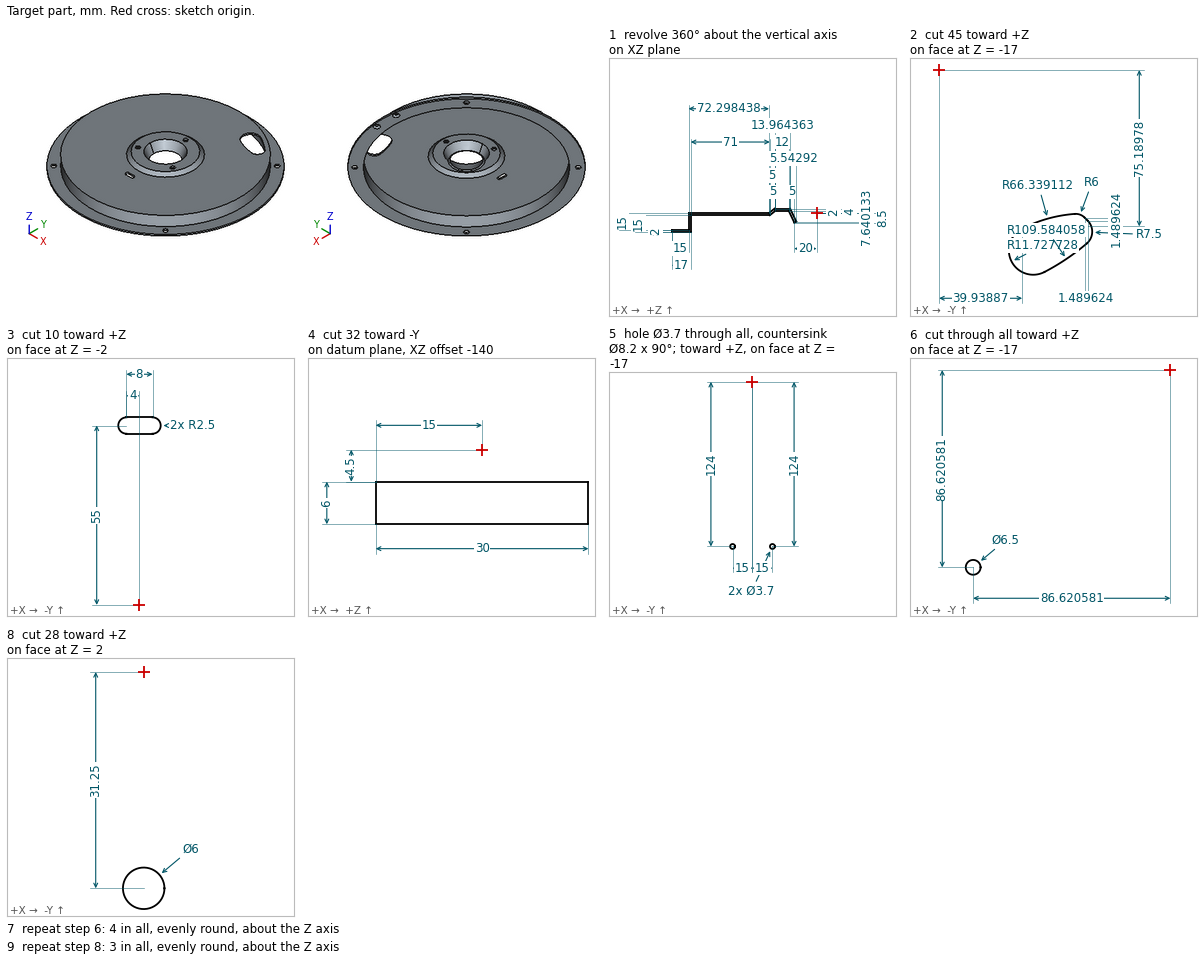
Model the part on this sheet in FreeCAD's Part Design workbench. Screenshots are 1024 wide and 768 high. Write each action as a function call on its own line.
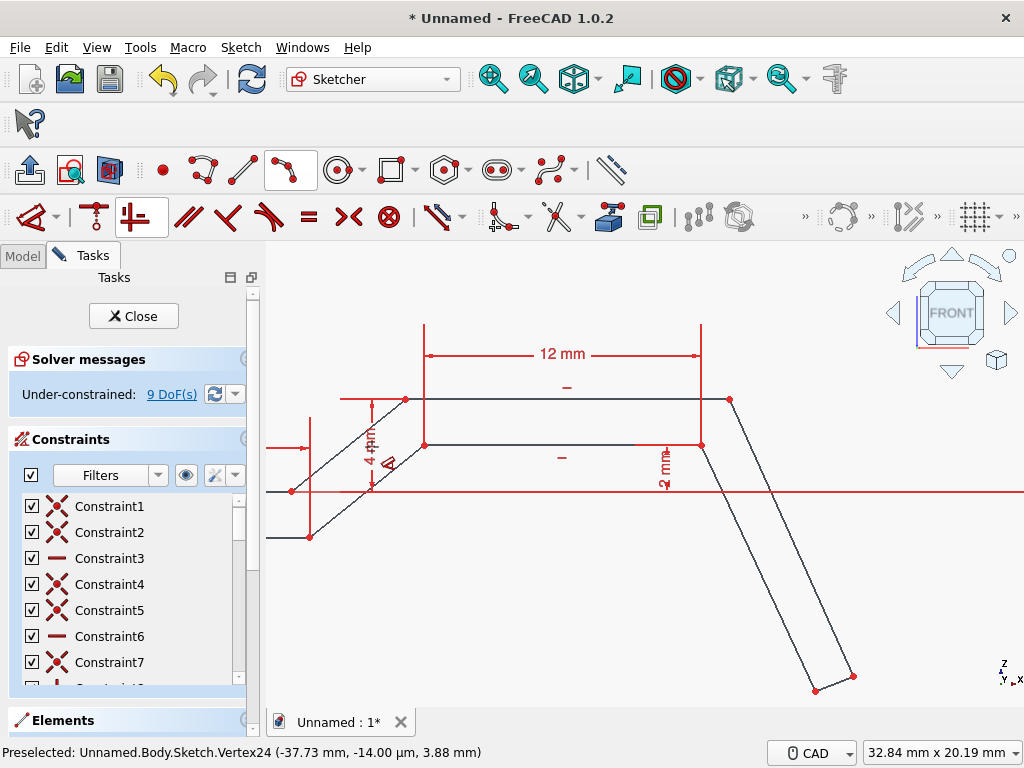
scroll(702, 448, down, 10)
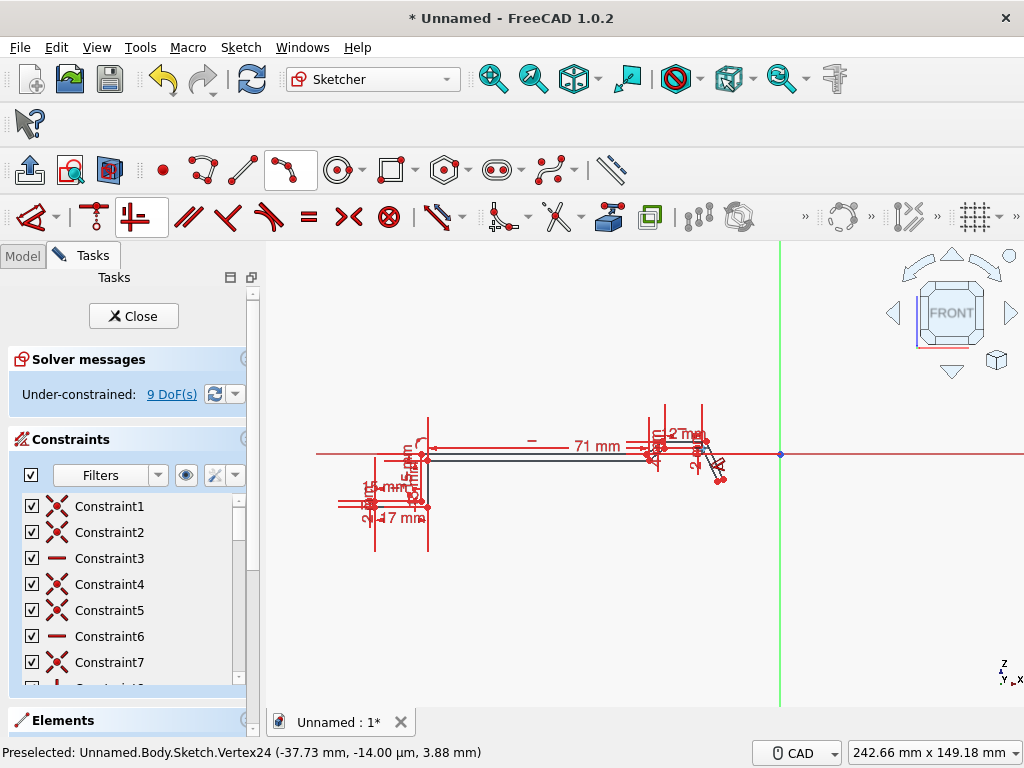
scroll(713, 471, up, 5)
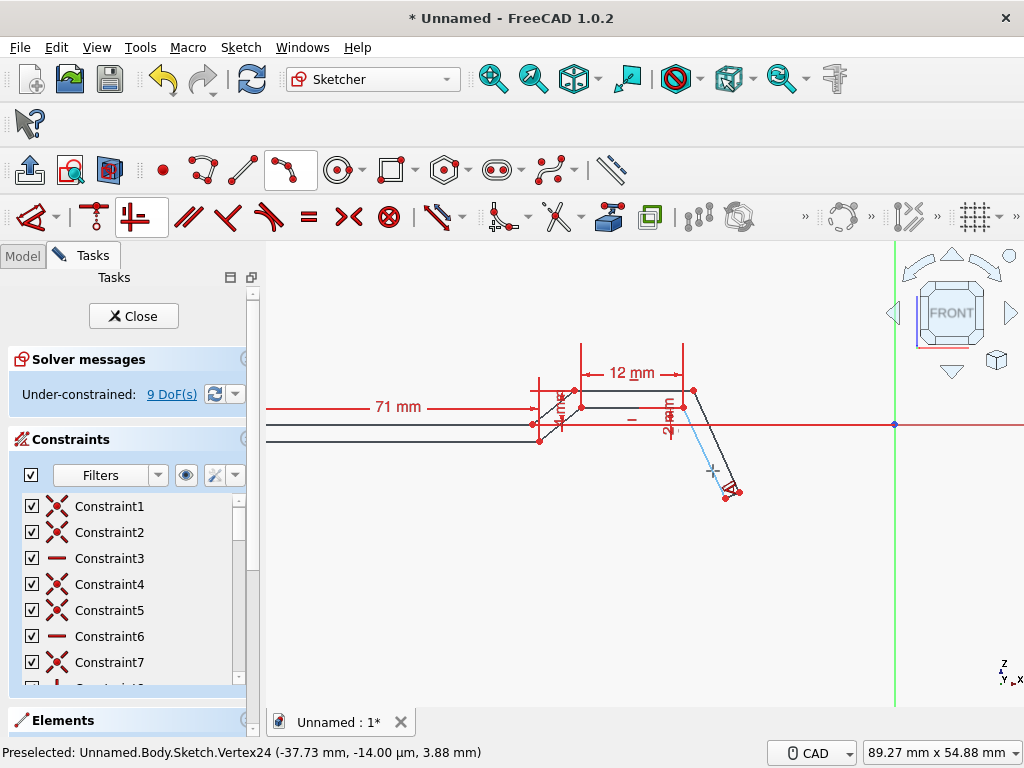
click(713, 471)
click(704, 374)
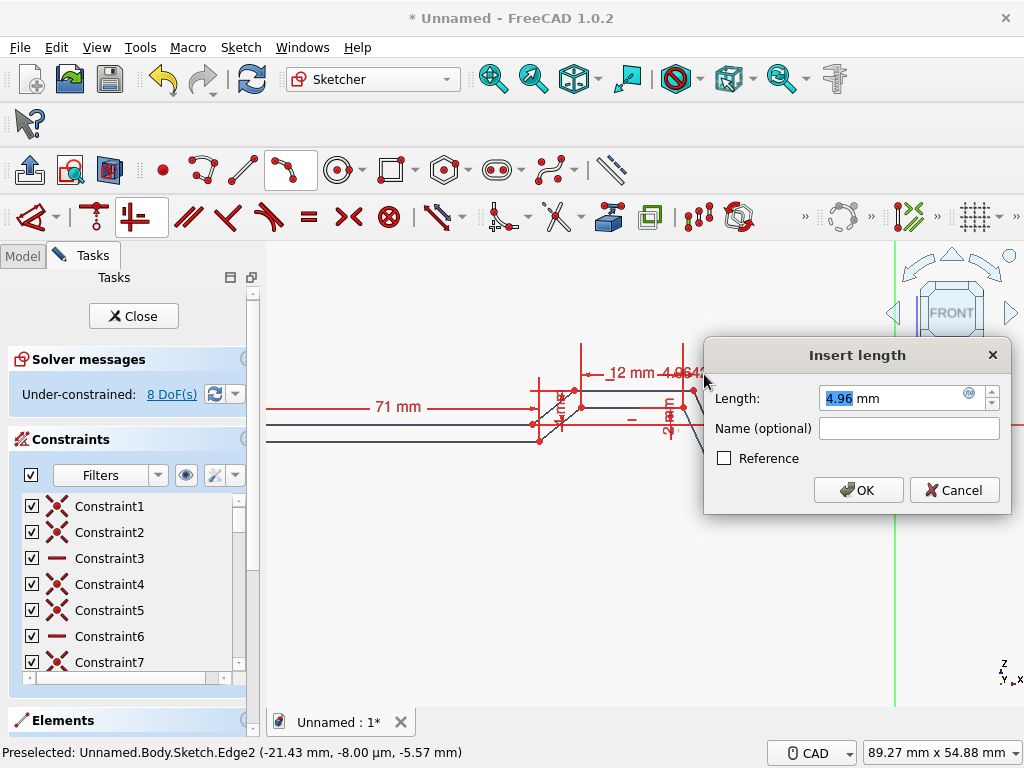
text(5)
key(Return)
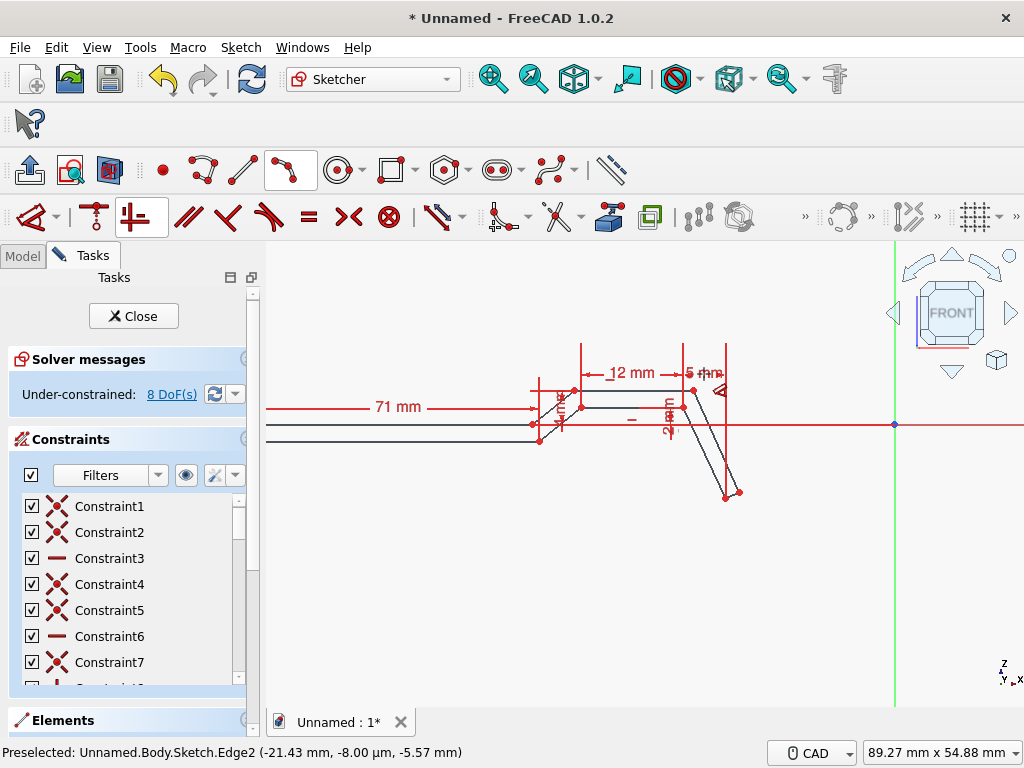
click(564, 421)
click(560, 374)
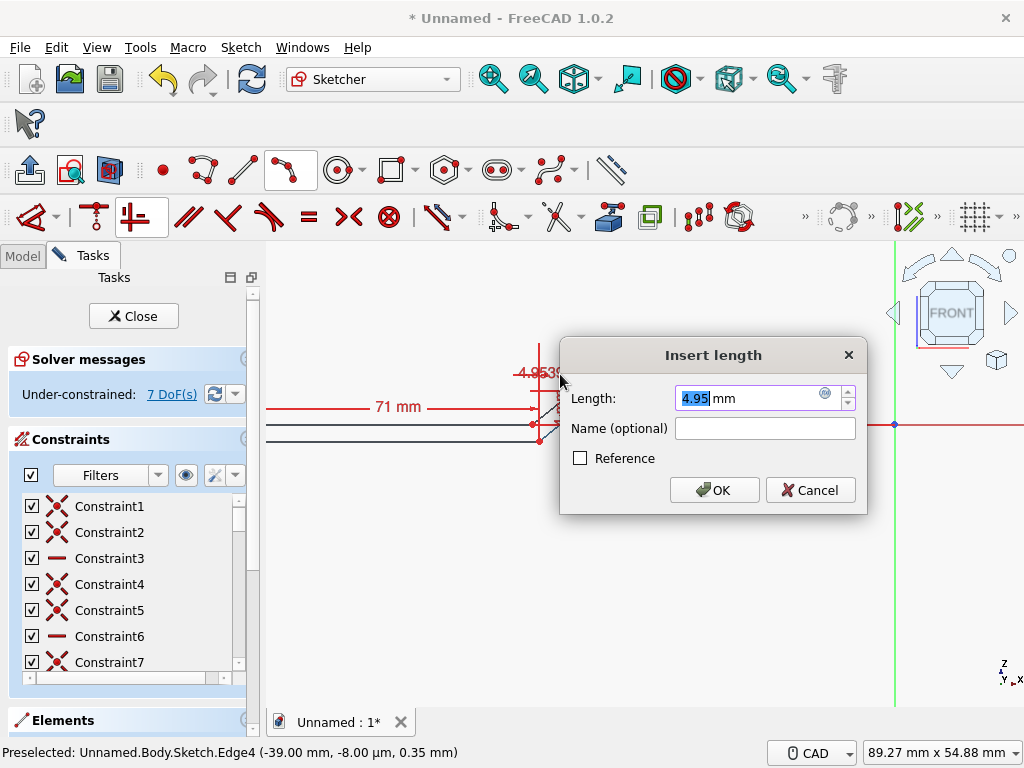
text(5)
key(Return)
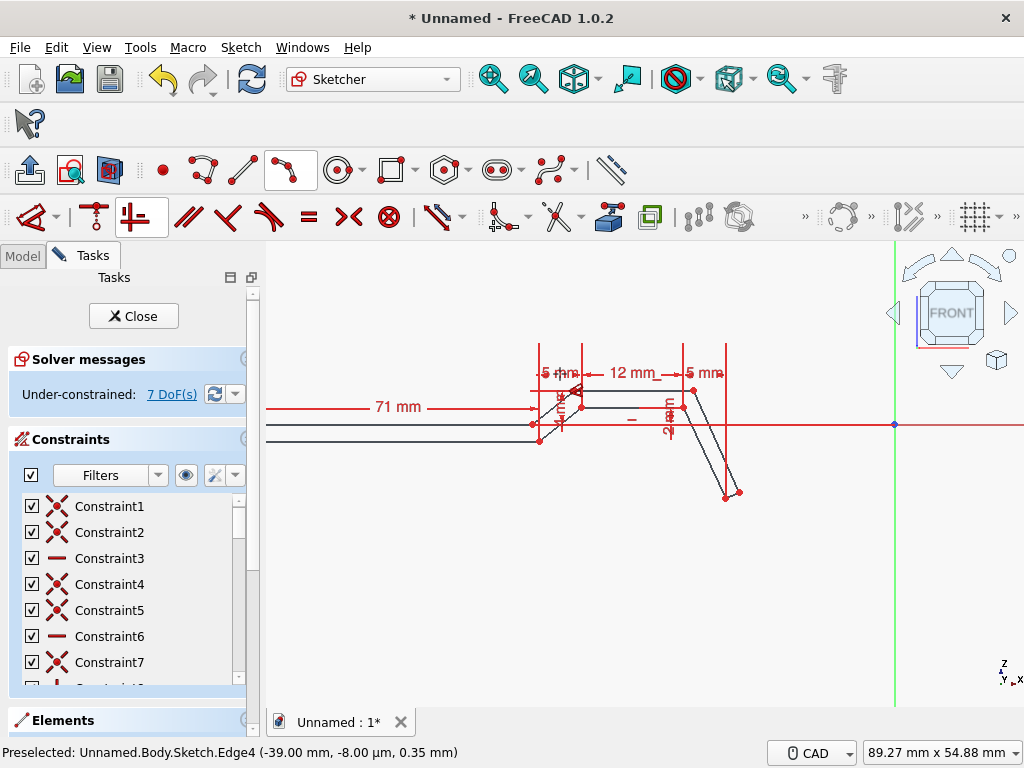
scroll(545, 415, up, 2)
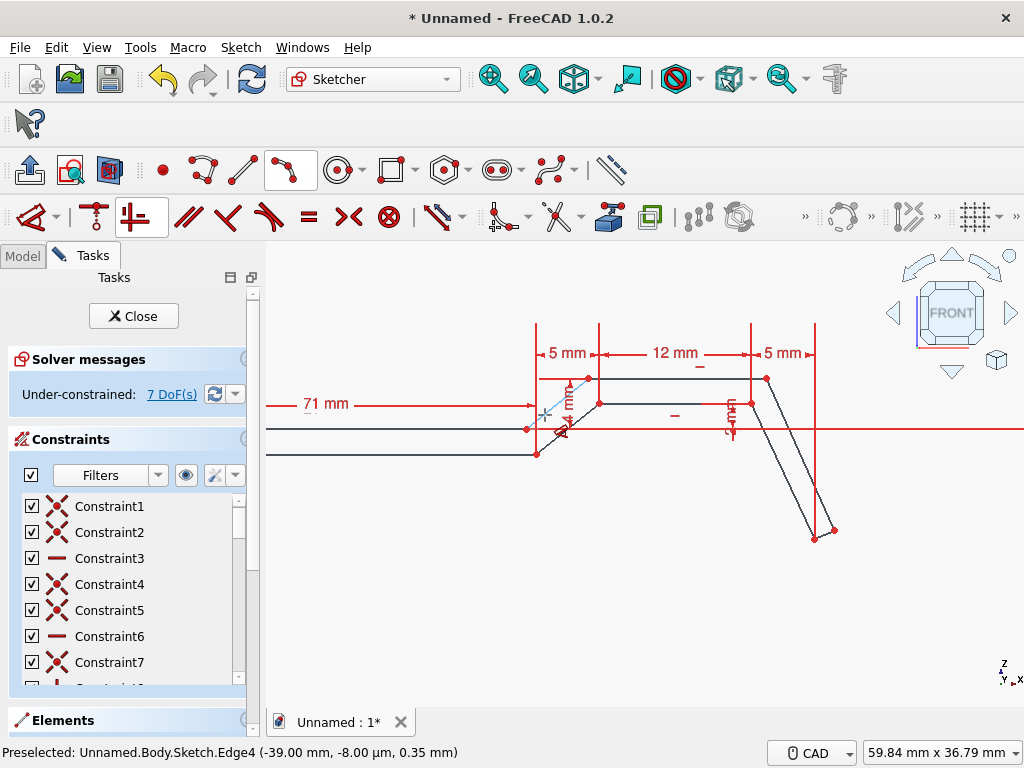
click(545, 414)
click(558, 463)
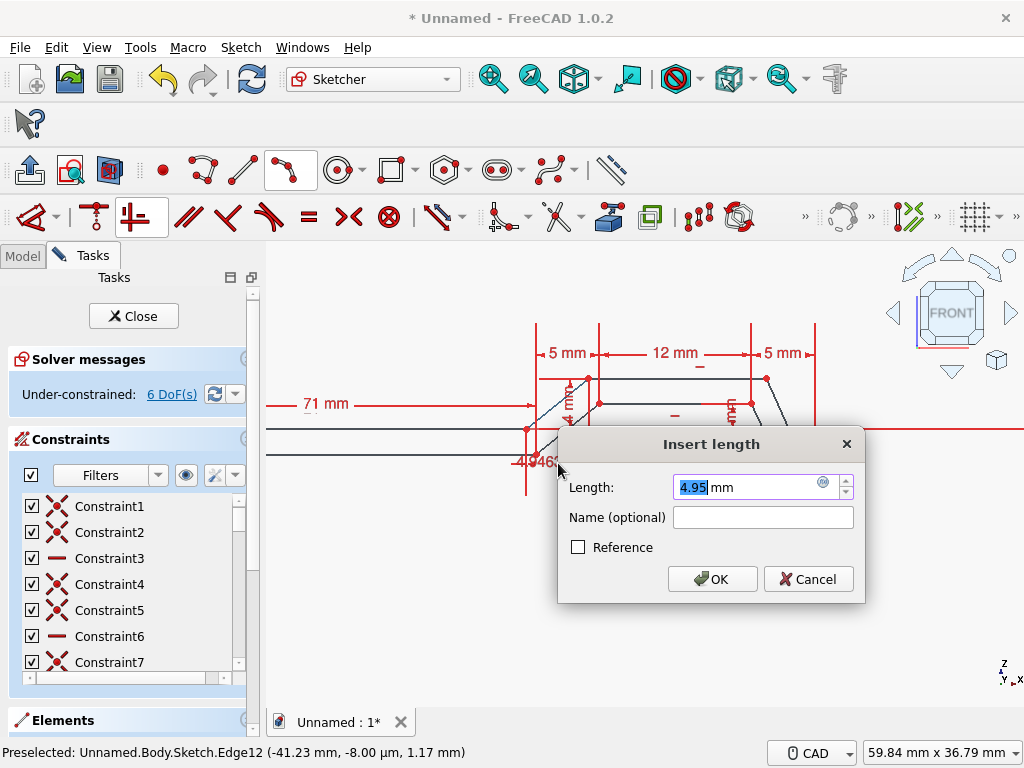
text(5)
key(Return)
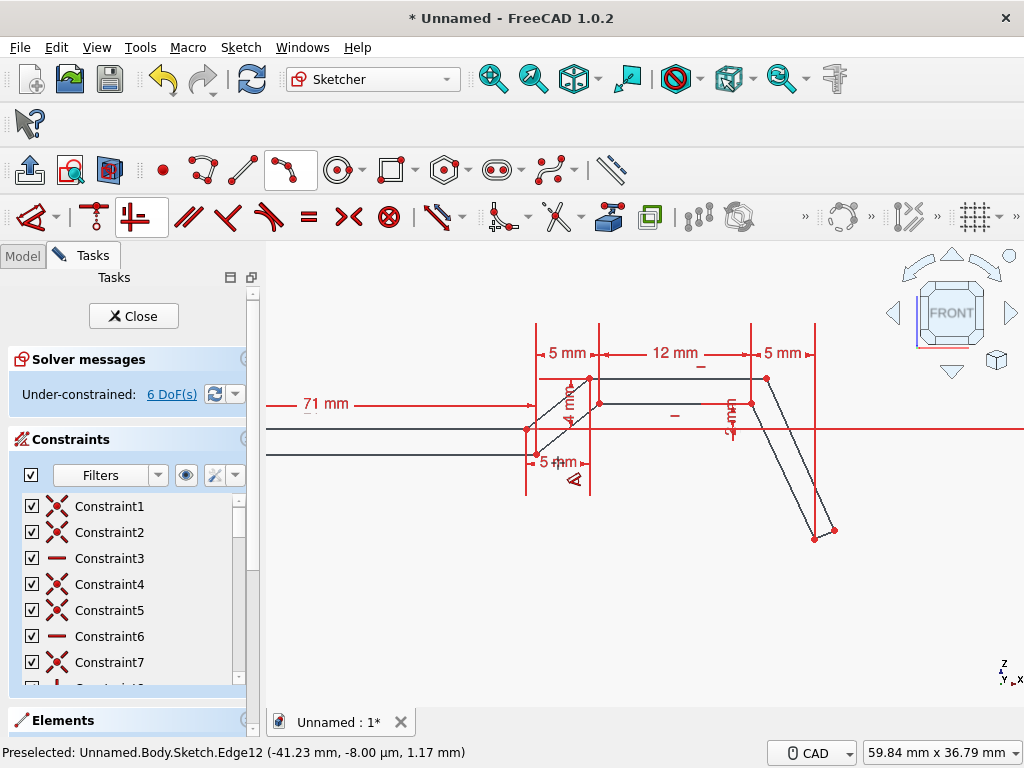
click(815, 539)
click(837, 395)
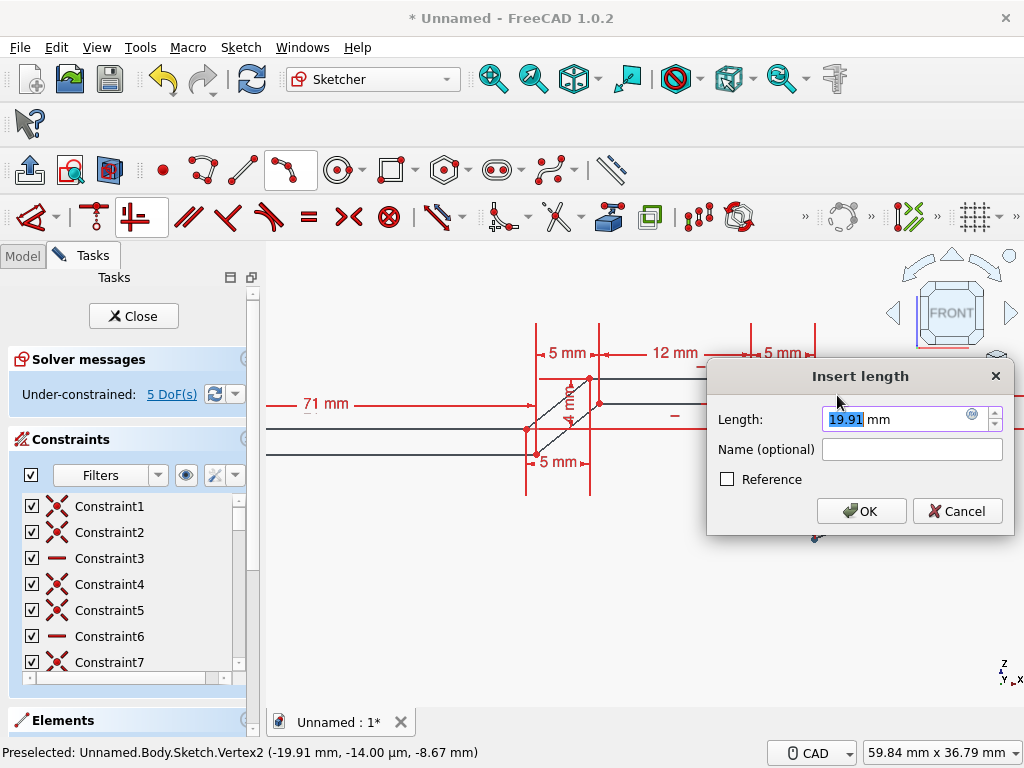
text(20)
key(Return)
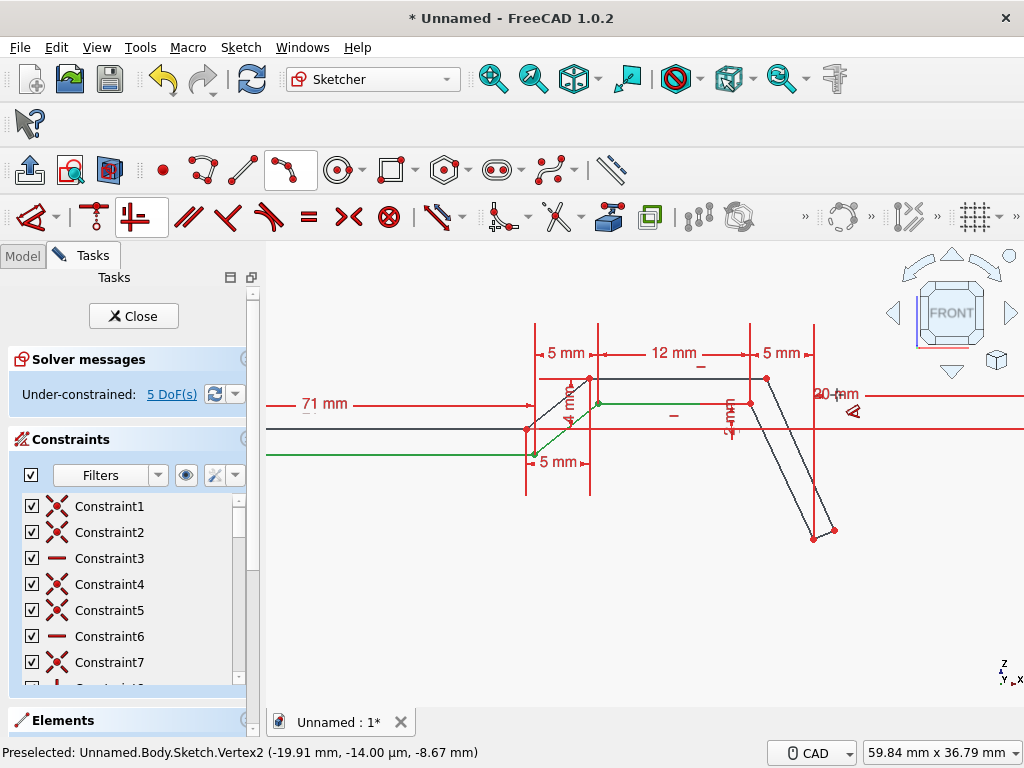
click(814, 539)
click(780, 509)